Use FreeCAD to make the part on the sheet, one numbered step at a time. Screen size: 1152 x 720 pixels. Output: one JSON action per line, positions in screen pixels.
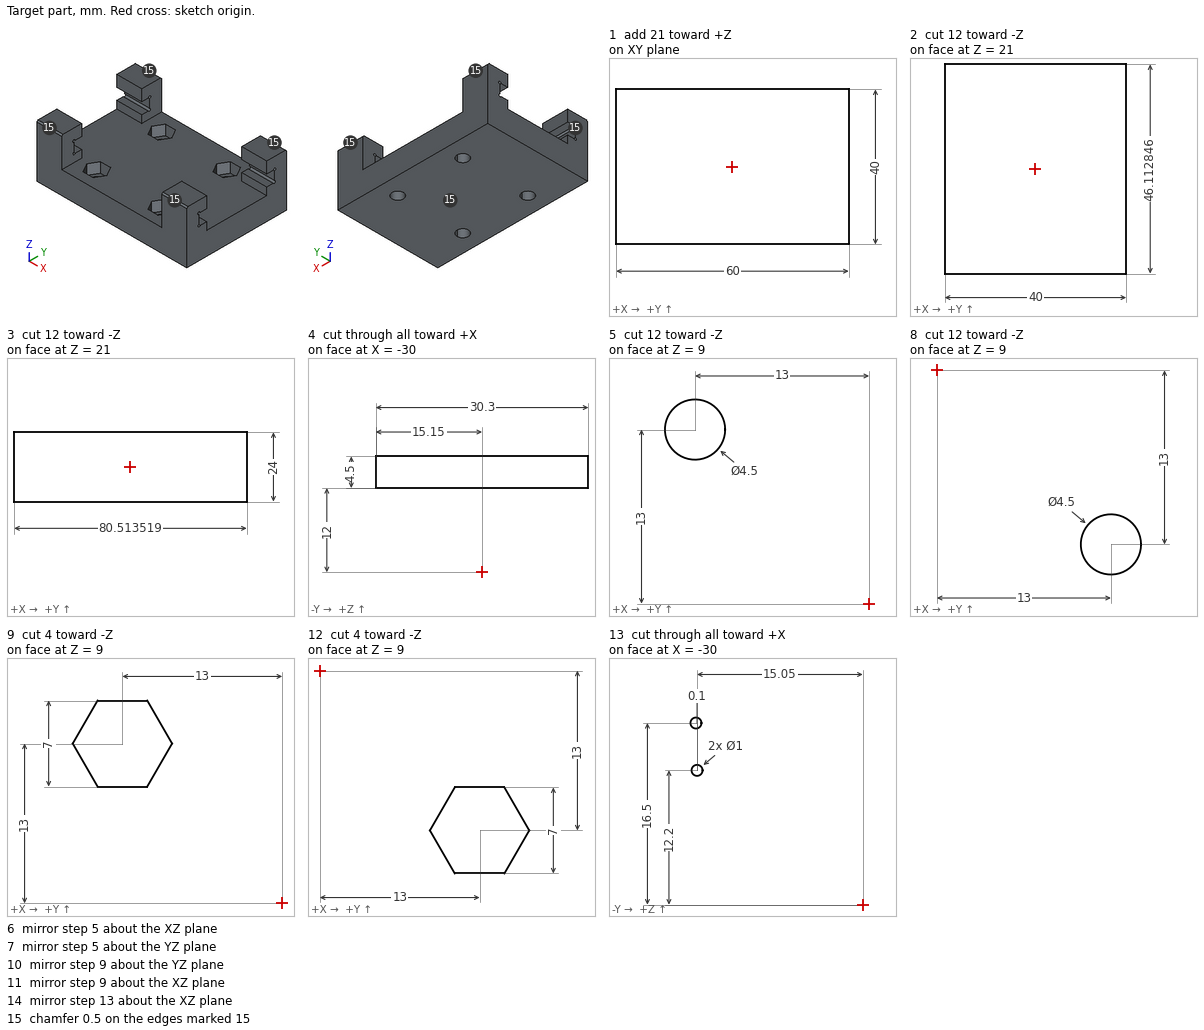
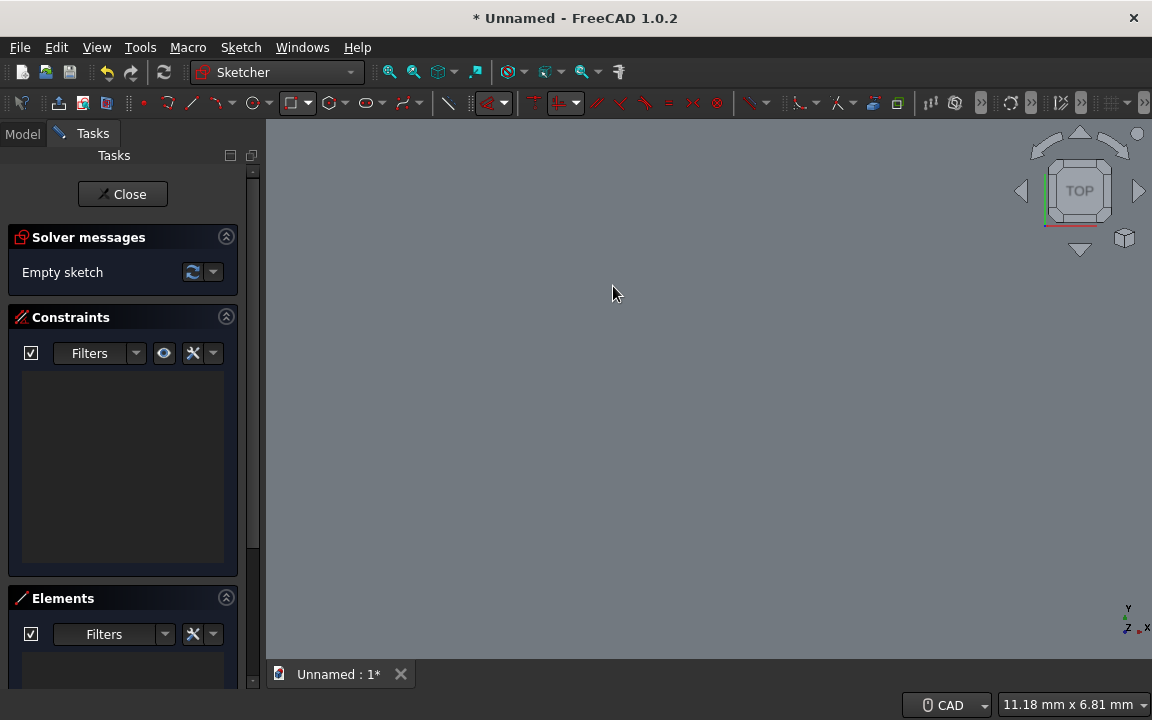
{"action": "left_click", "coordinate": [254, 104]}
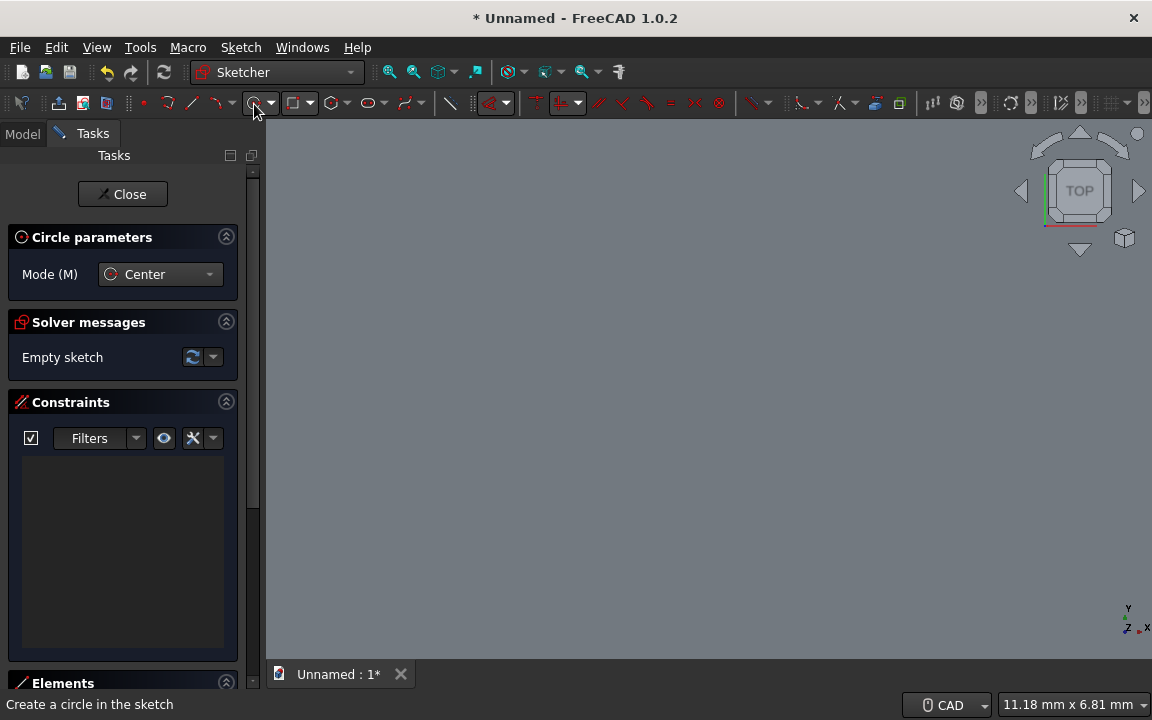
{"action": "left_click", "coordinate": [637, 388]}
{"action": "left_click", "coordinate": [763, 262]}
{"action": "key", "text": "Escape"}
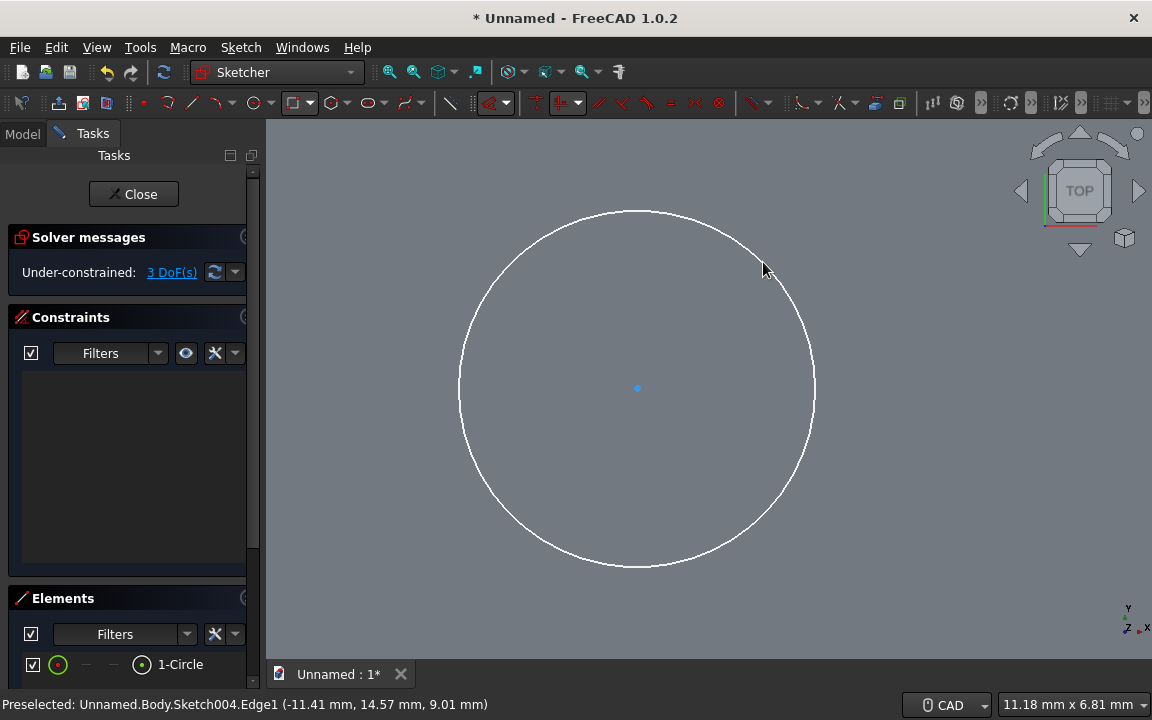
{"action": "left_click", "coordinate": [763, 263]}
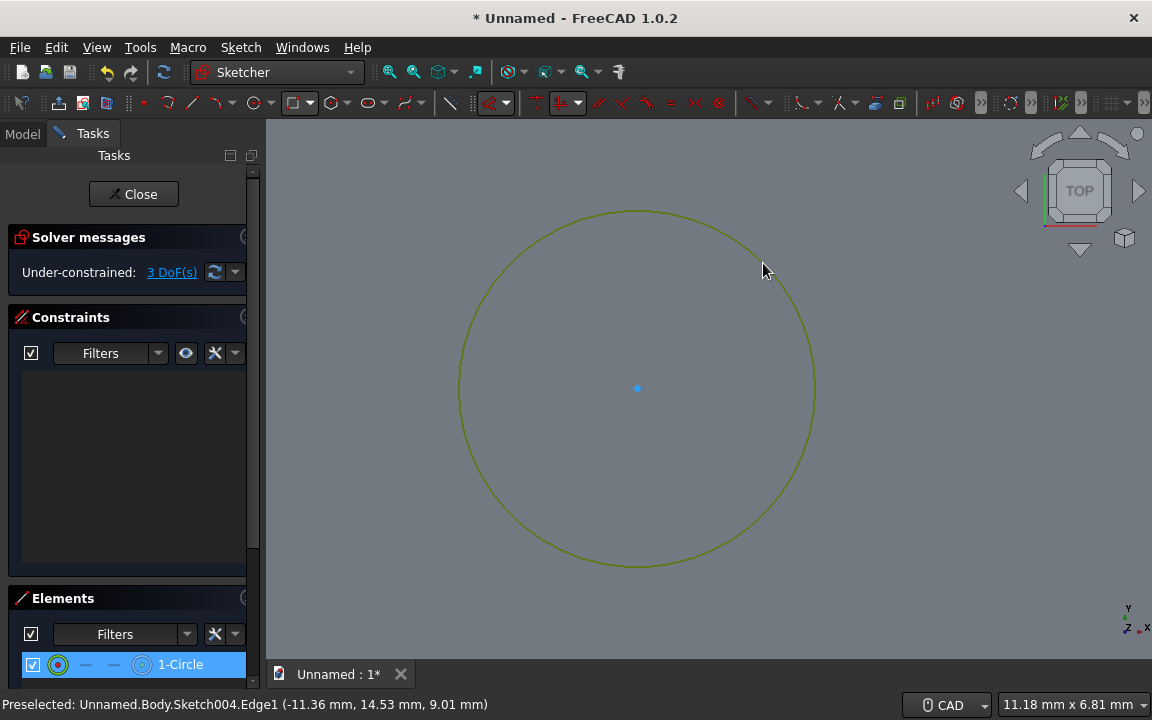
{"action": "left_click", "coordinate": [508, 104]}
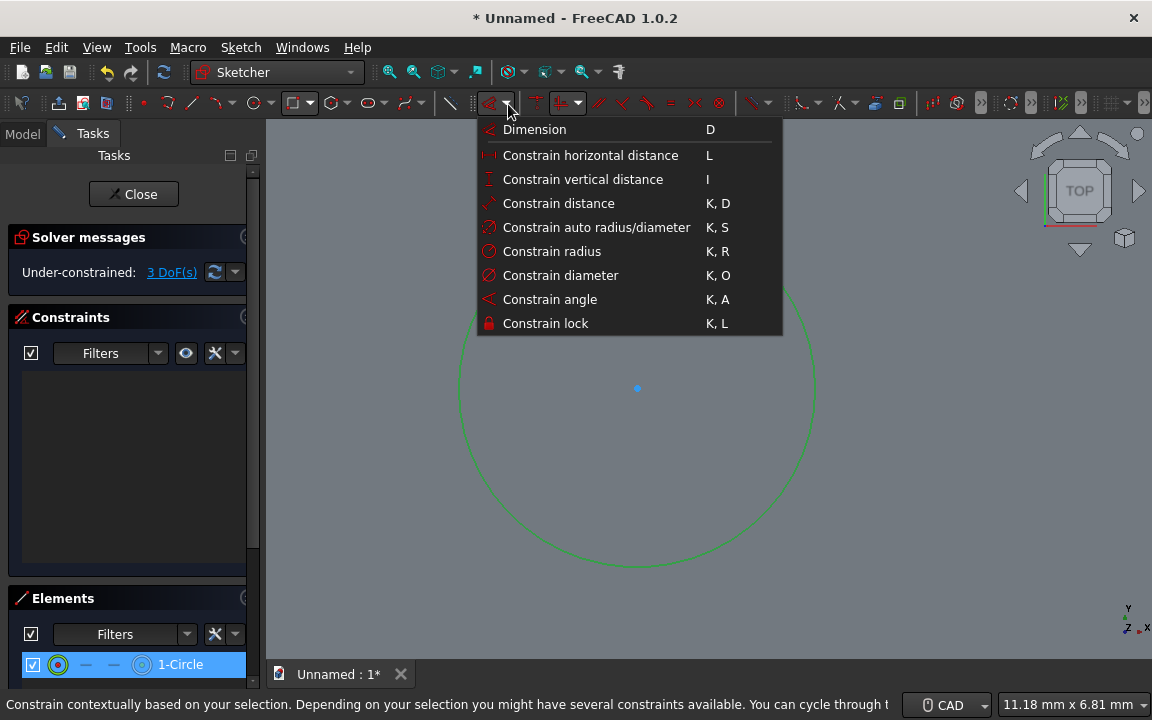
{"action": "left_click", "coordinate": [630, 275]}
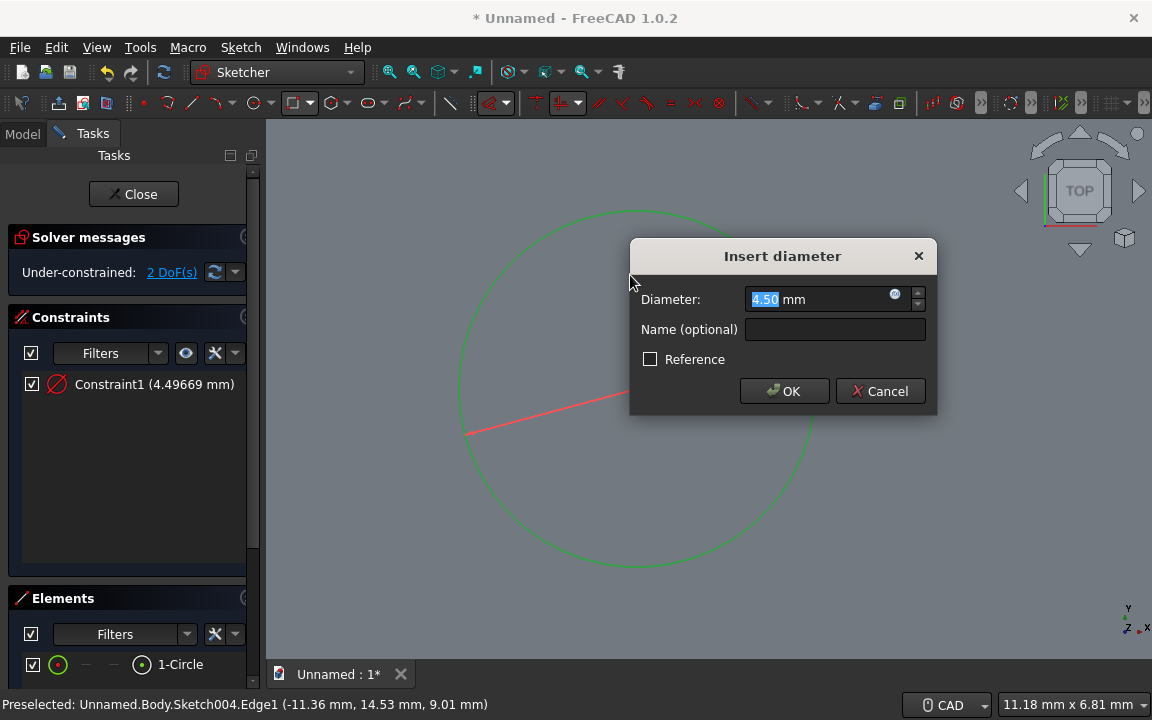
{"action": "type", "text": "4.5"}
{"action": "key", "text": "Return"}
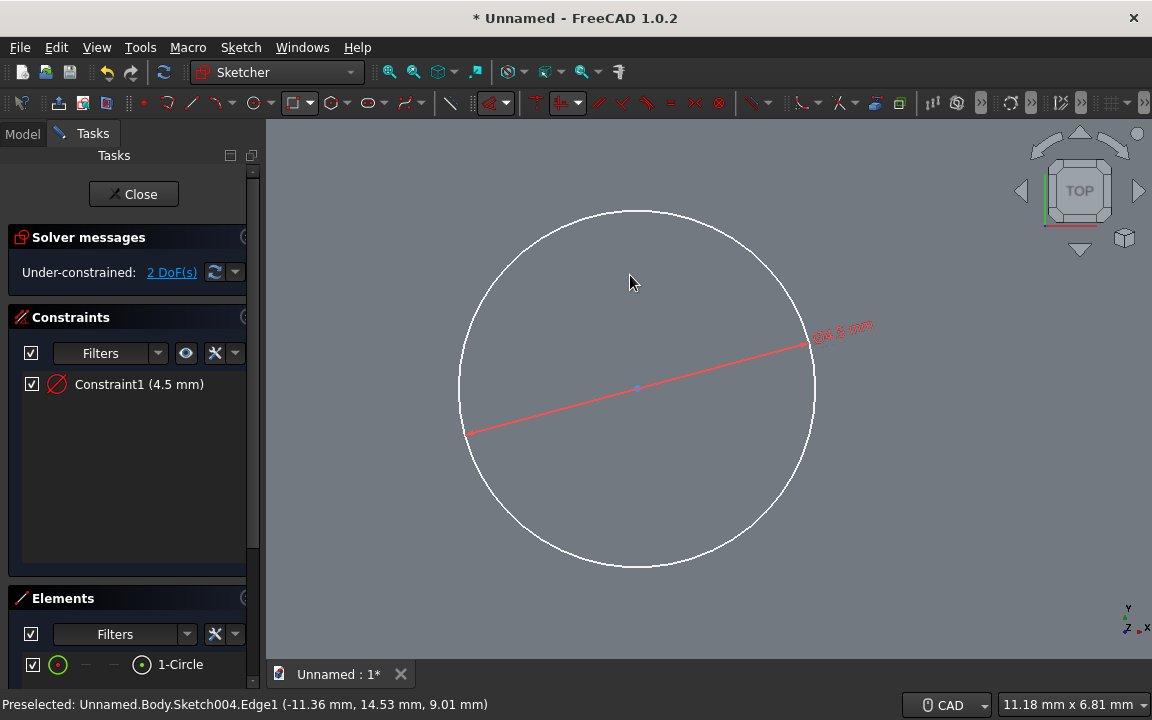
{"action": "left_click", "coordinate": [637, 389]}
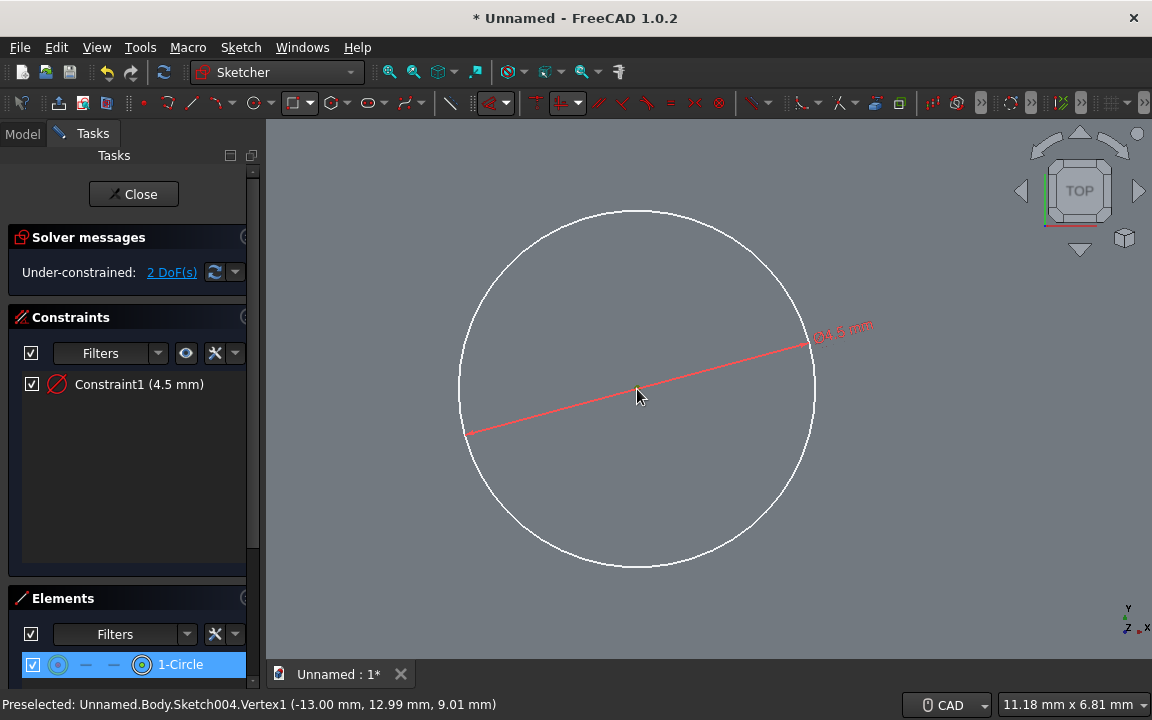
{"action": "key", "text": "l"}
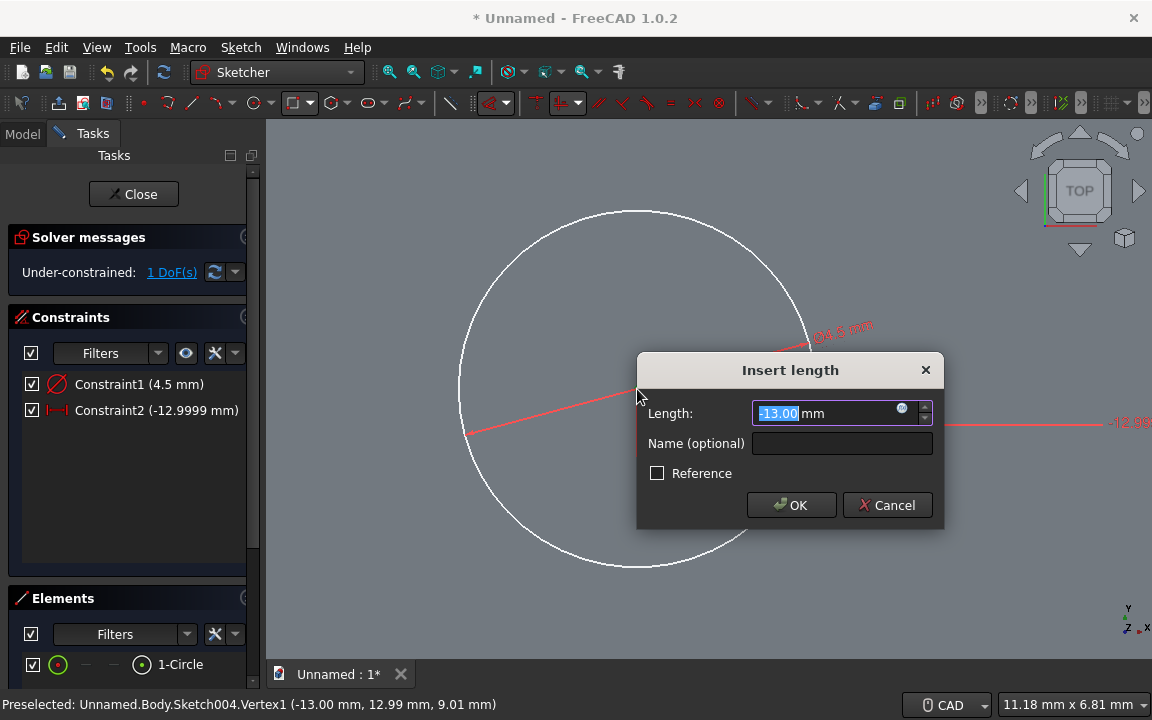
{"action": "type", "text": "-13"}
{"action": "key", "text": "Return"}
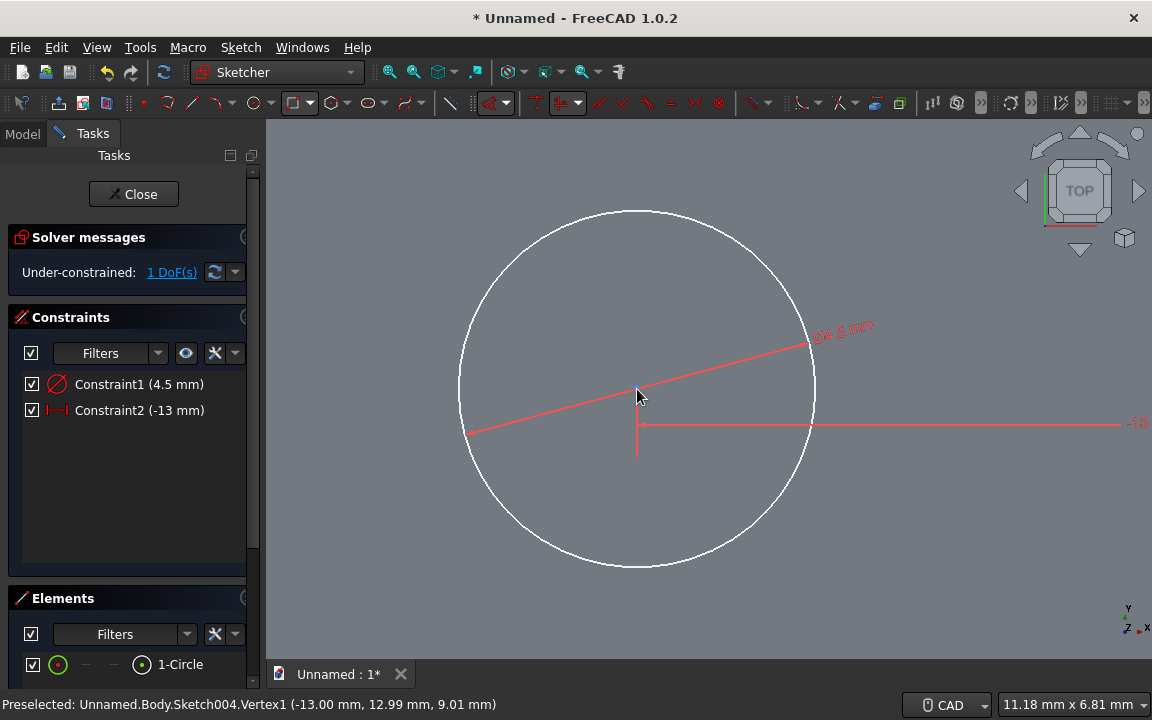
{"action": "left_click", "coordinate": [637, 389]}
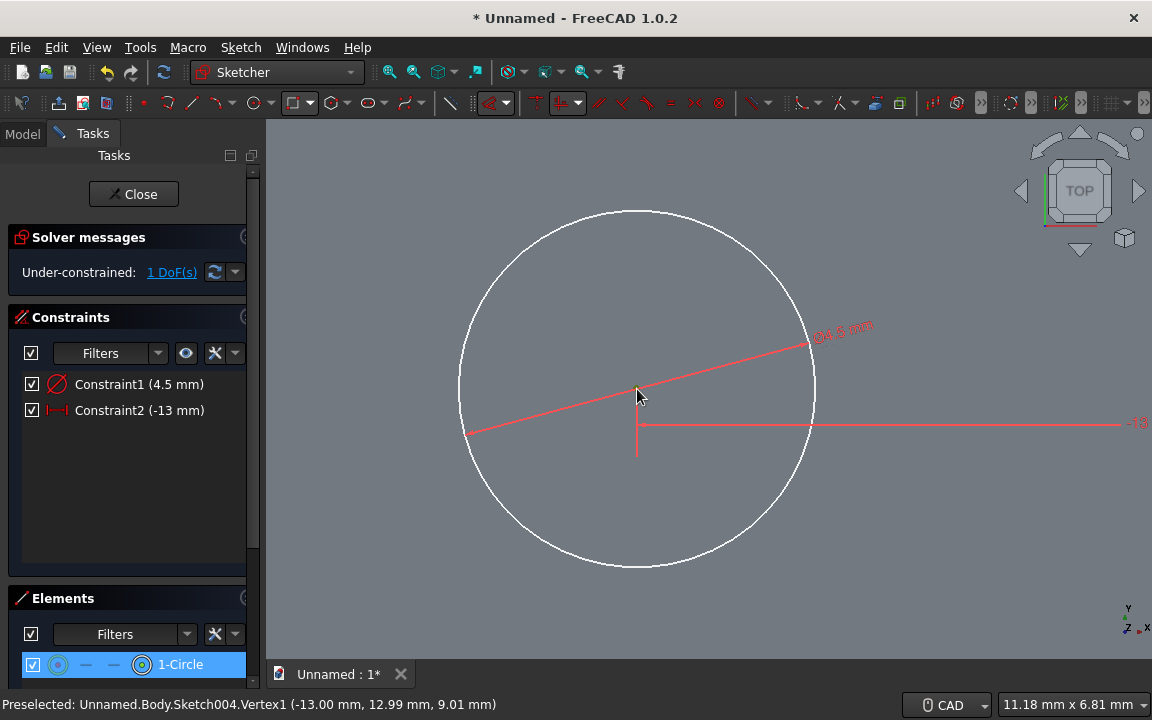
{"action": "left_click", "coordinate": [508, 104]}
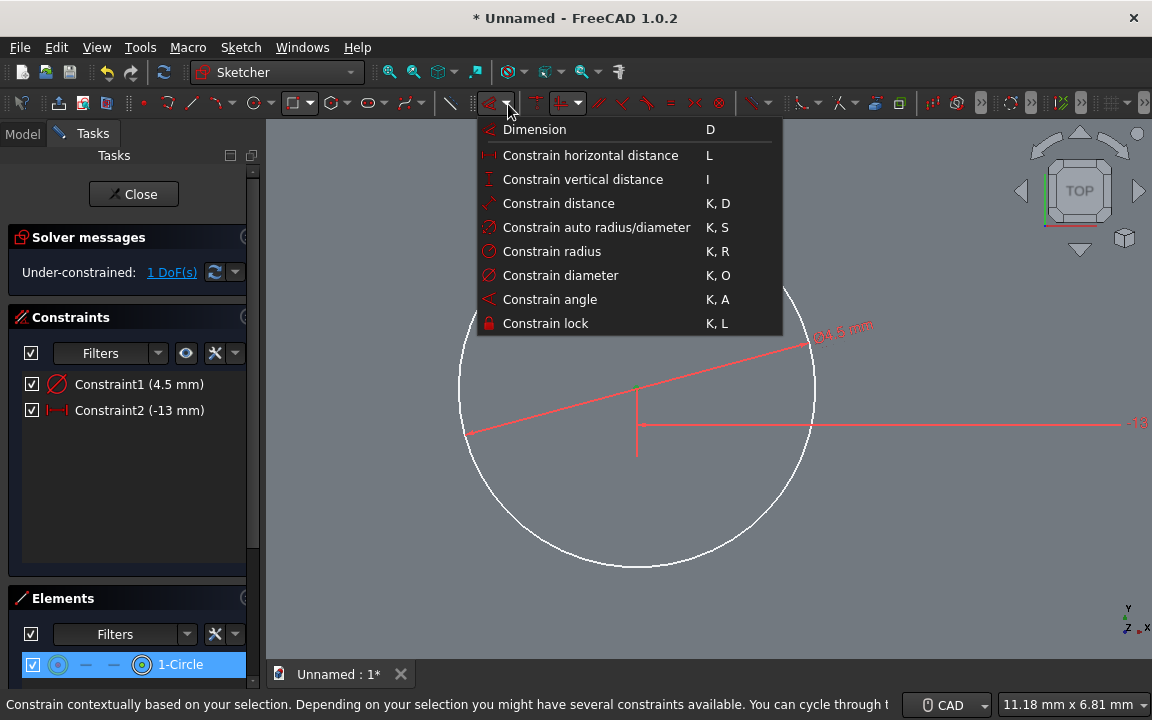
{"action": "left_click", "coordinate": [630, 179]}